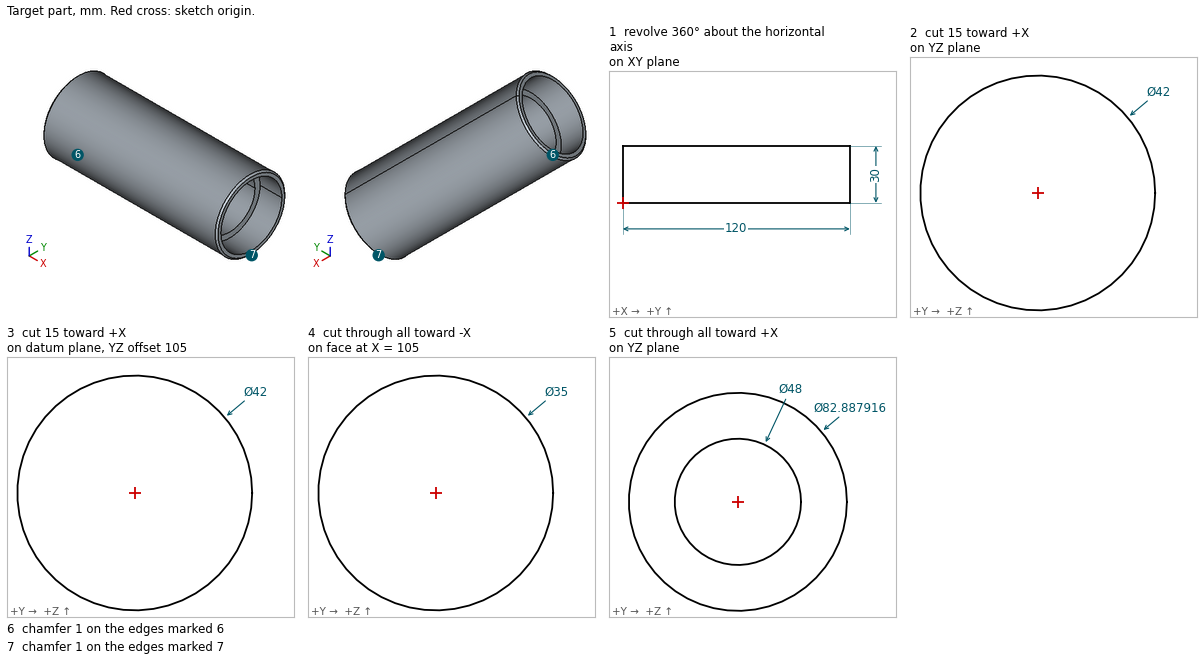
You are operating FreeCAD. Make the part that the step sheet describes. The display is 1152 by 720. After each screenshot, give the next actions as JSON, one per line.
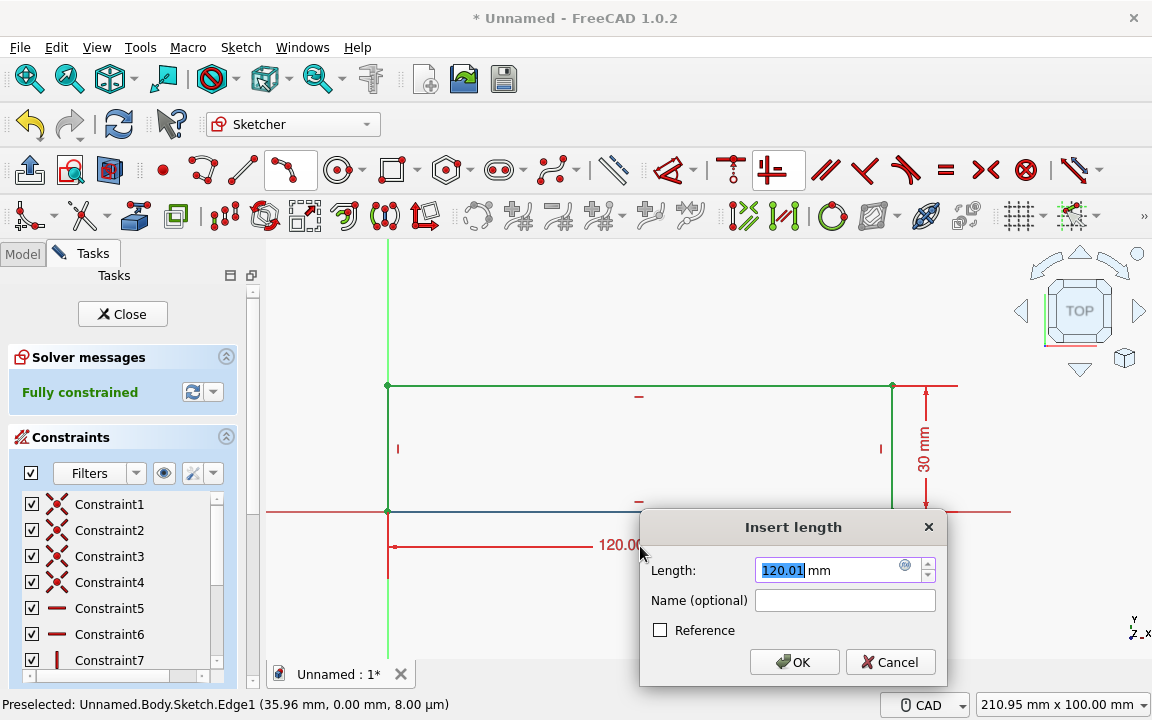
{"action": "type", "text": "120"}
{"action": "key", "text": "Return"}
{"action": "key", "text": "Escape"}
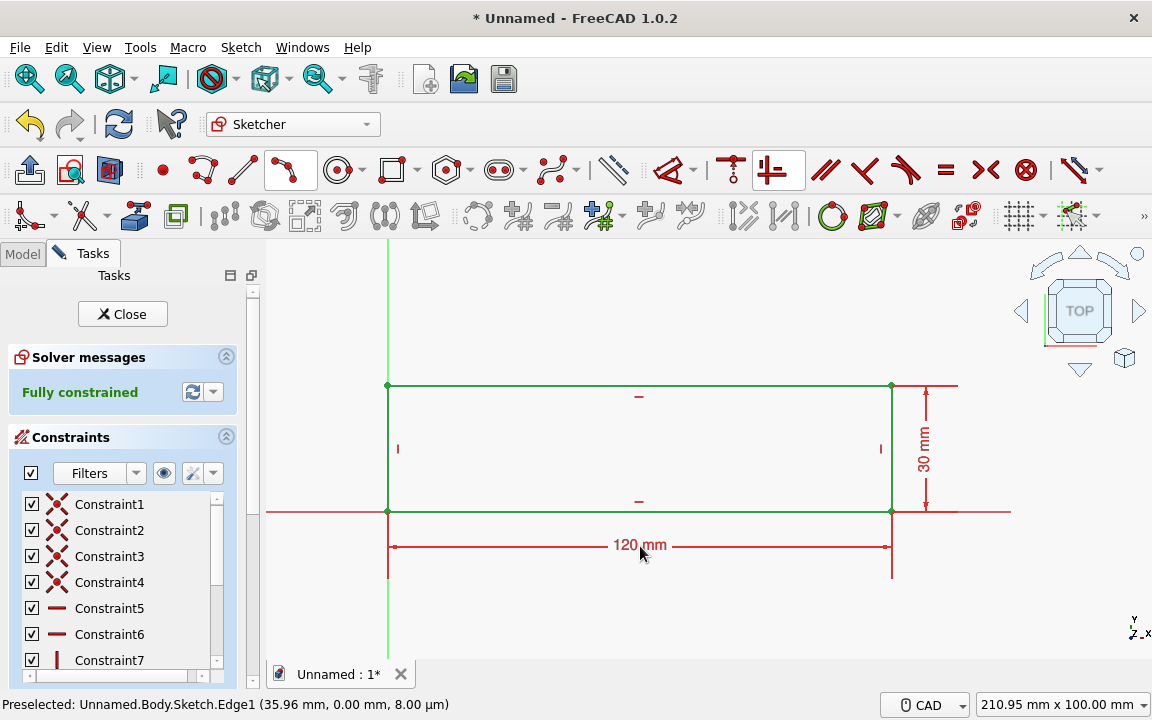
{"action": "left_click", "coordinate": [123, 314]}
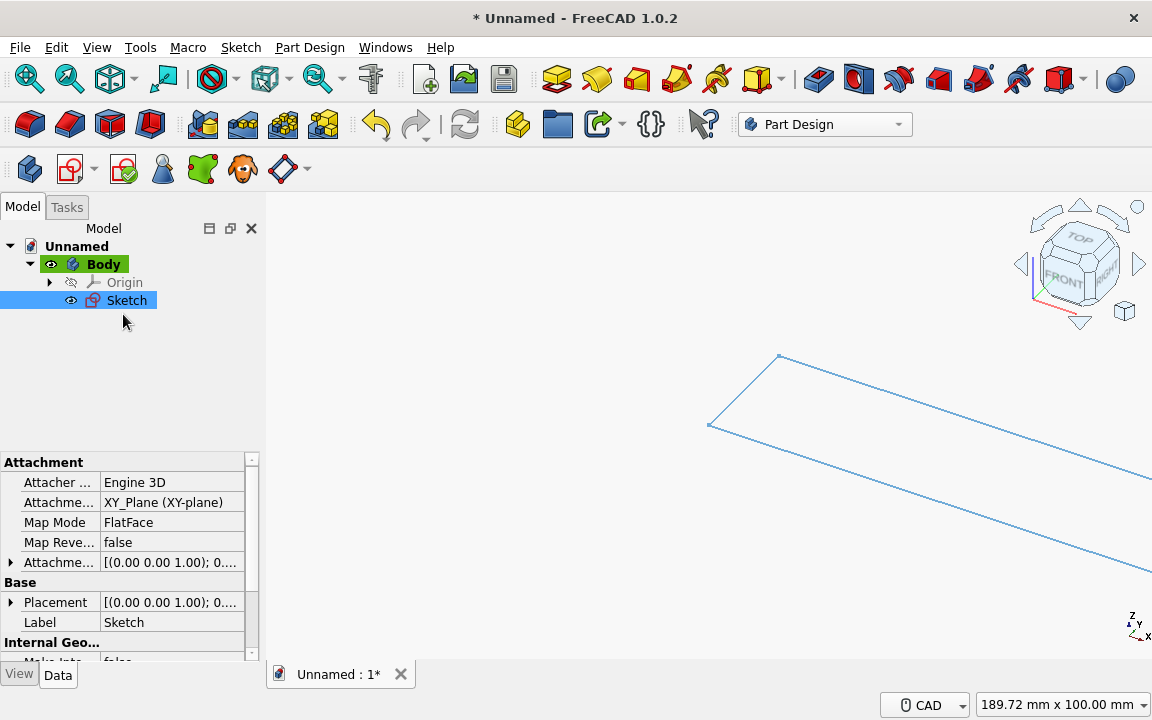
{"action": "left_click", "coordinate": [598, 80]}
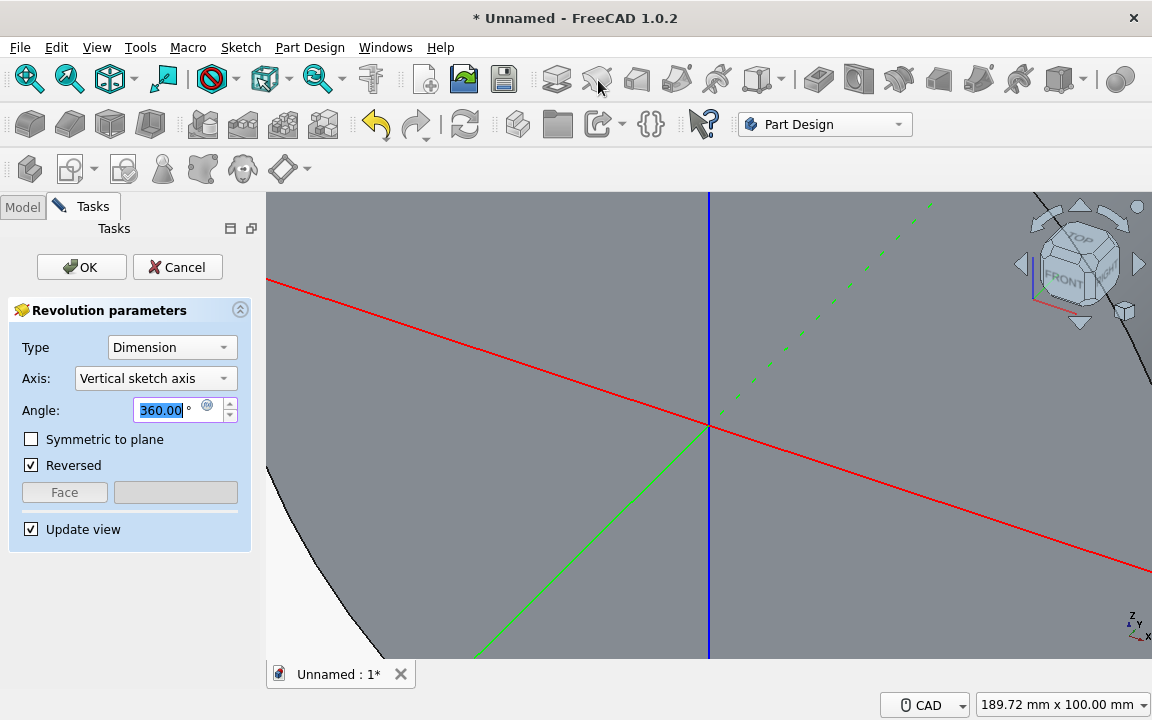
{"action": "left_click", "coordinate": [156, 378]}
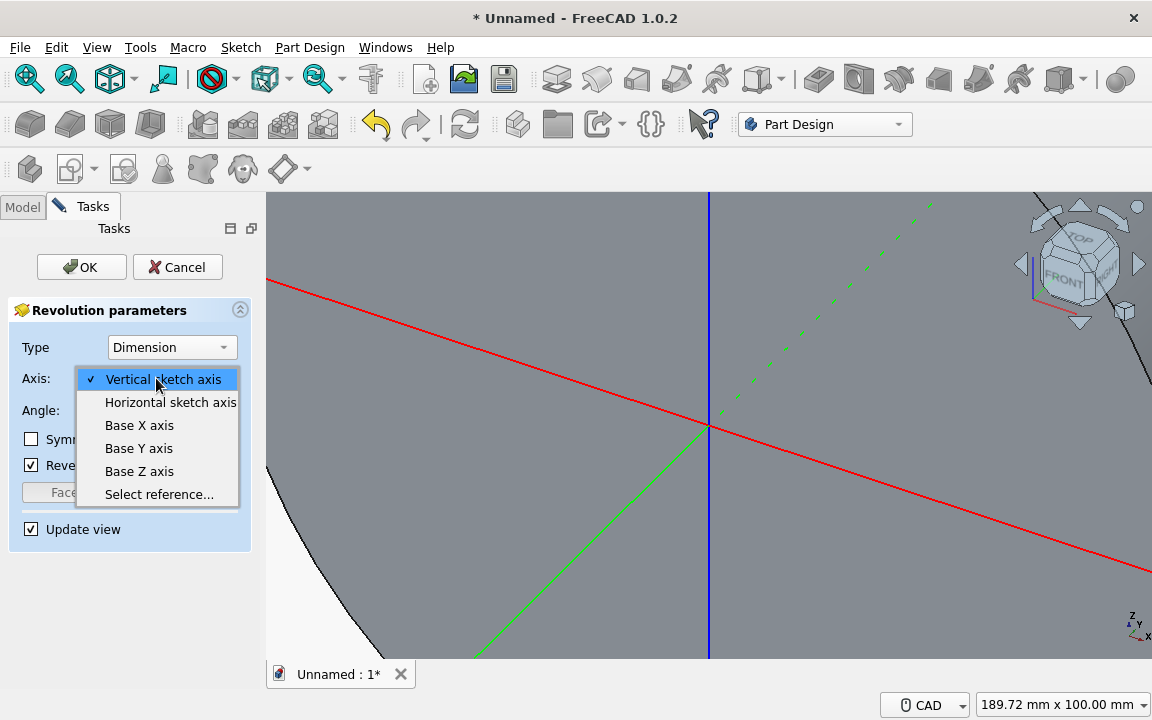
{"action": "left_click", "coordinate": [156, 402]}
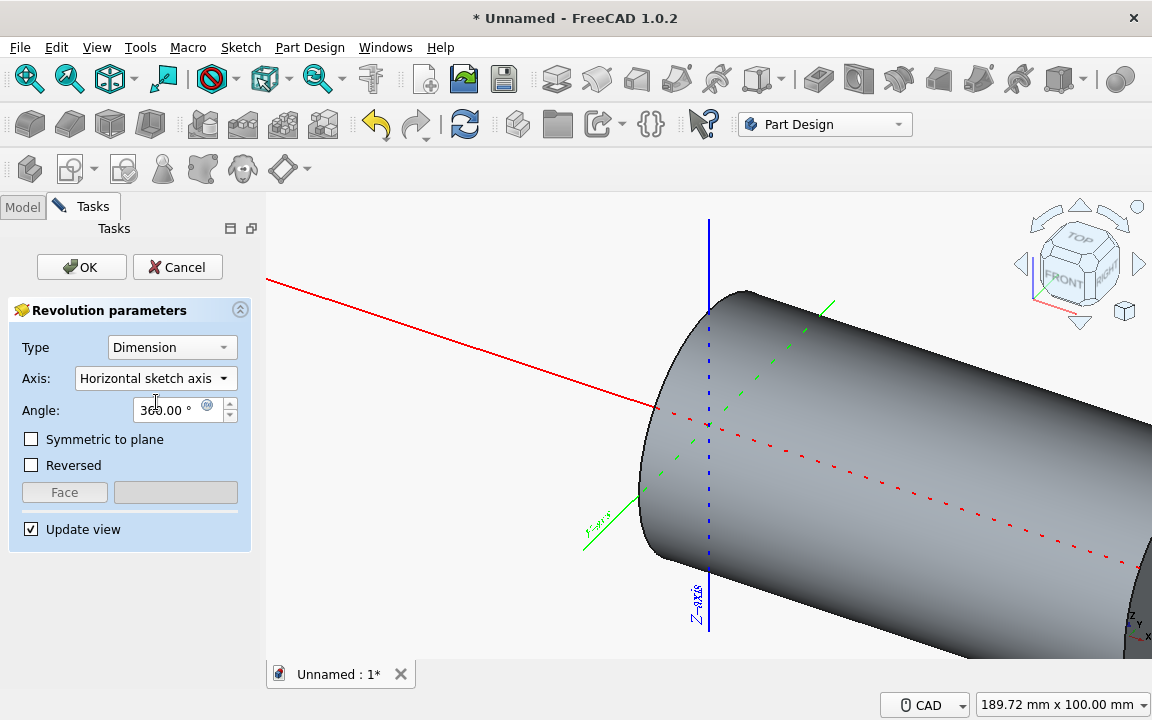
{"action": "left_click", "coordinate": [82, 267]}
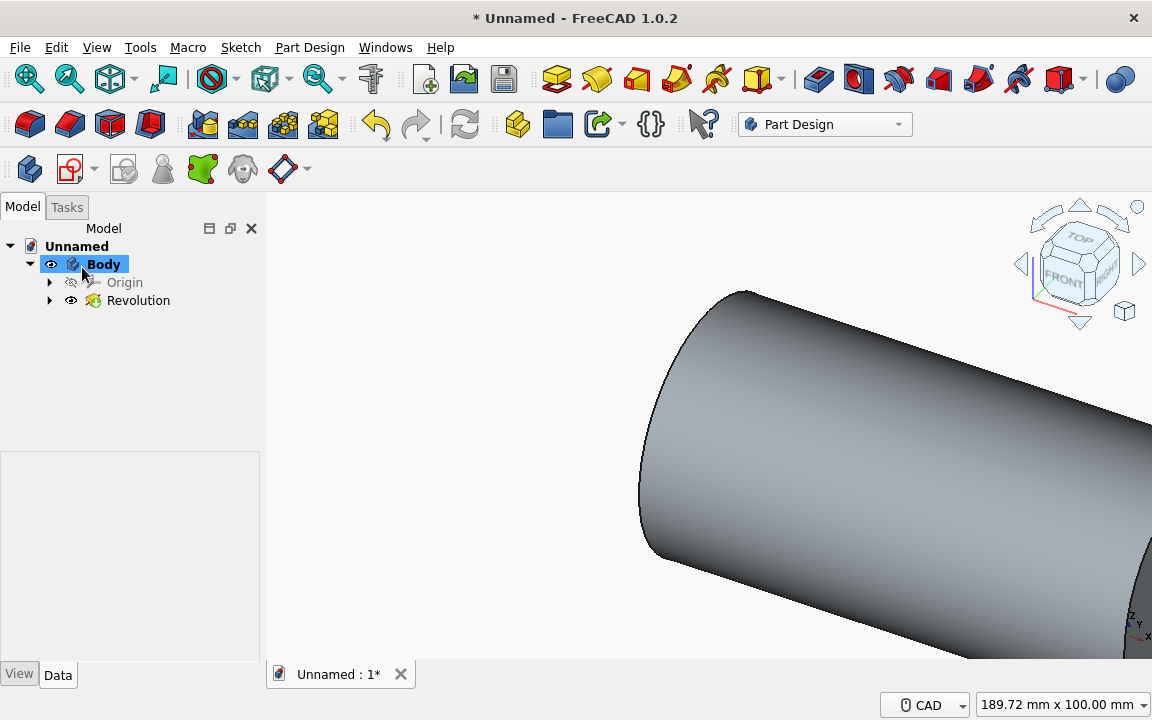
{"action": "key", "text": "v f"}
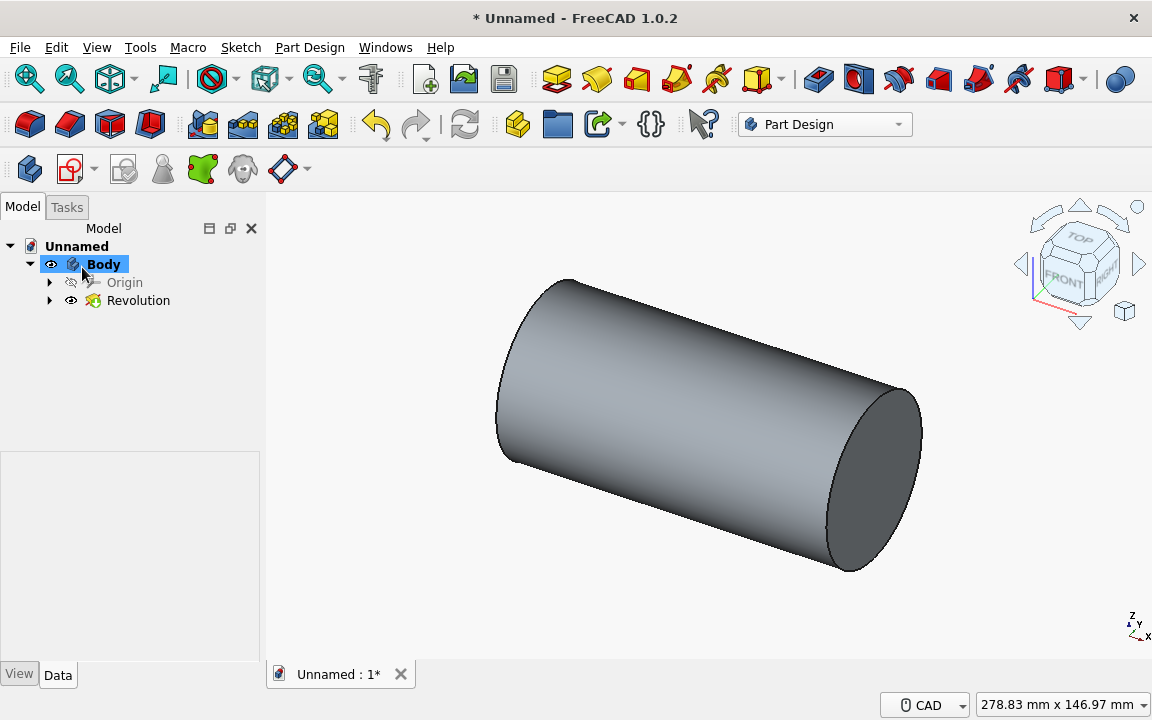
{"action": "left_click", "coordinate": [70, 170]}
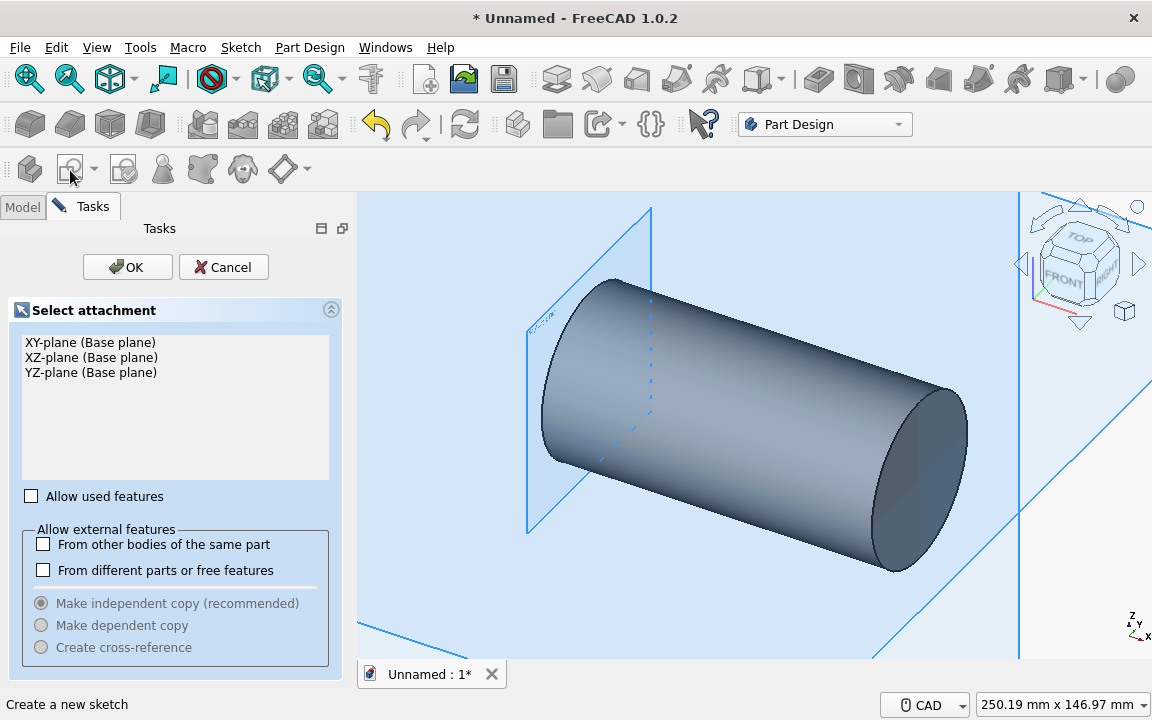
{"action": "left_click", "coordinate": [82, 372]}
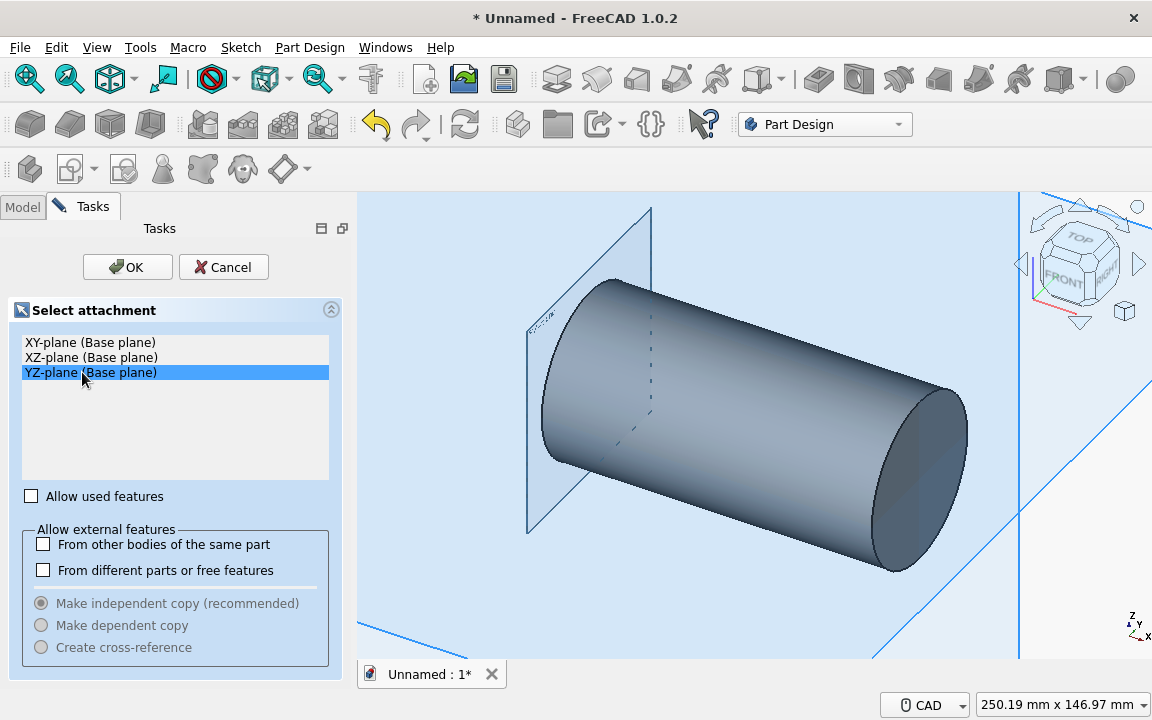
{"action": "left_click", "coordinate": [128, 267]}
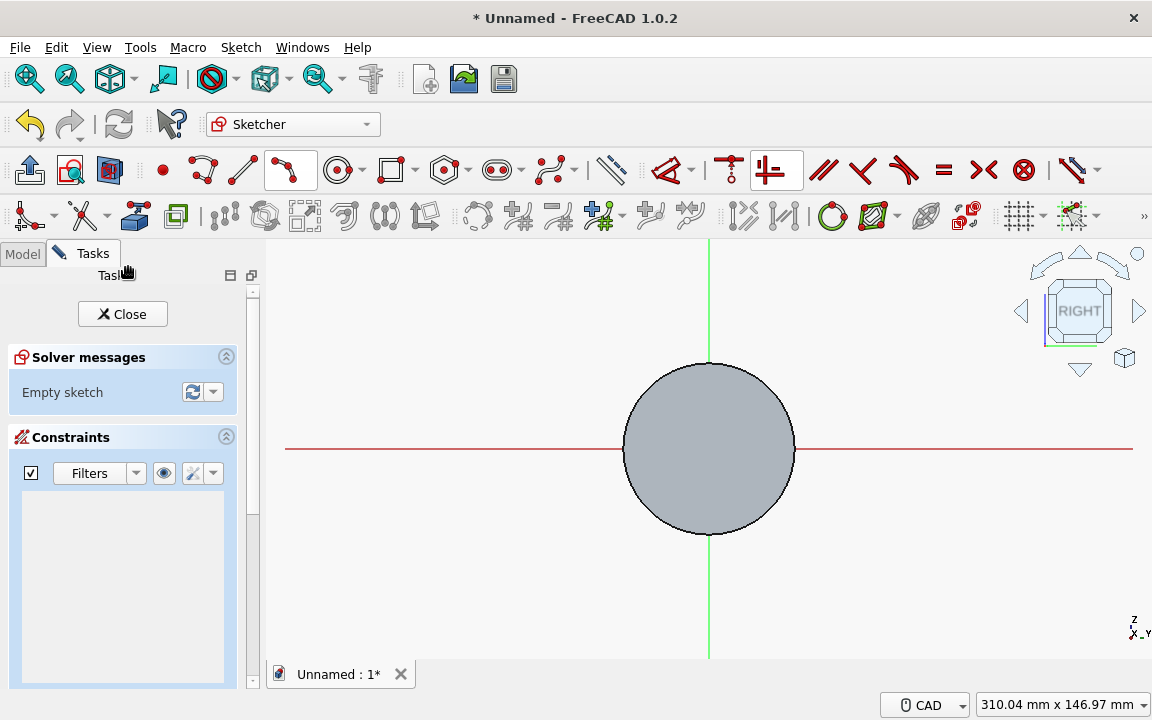
{"action": "key", "text": "q s"}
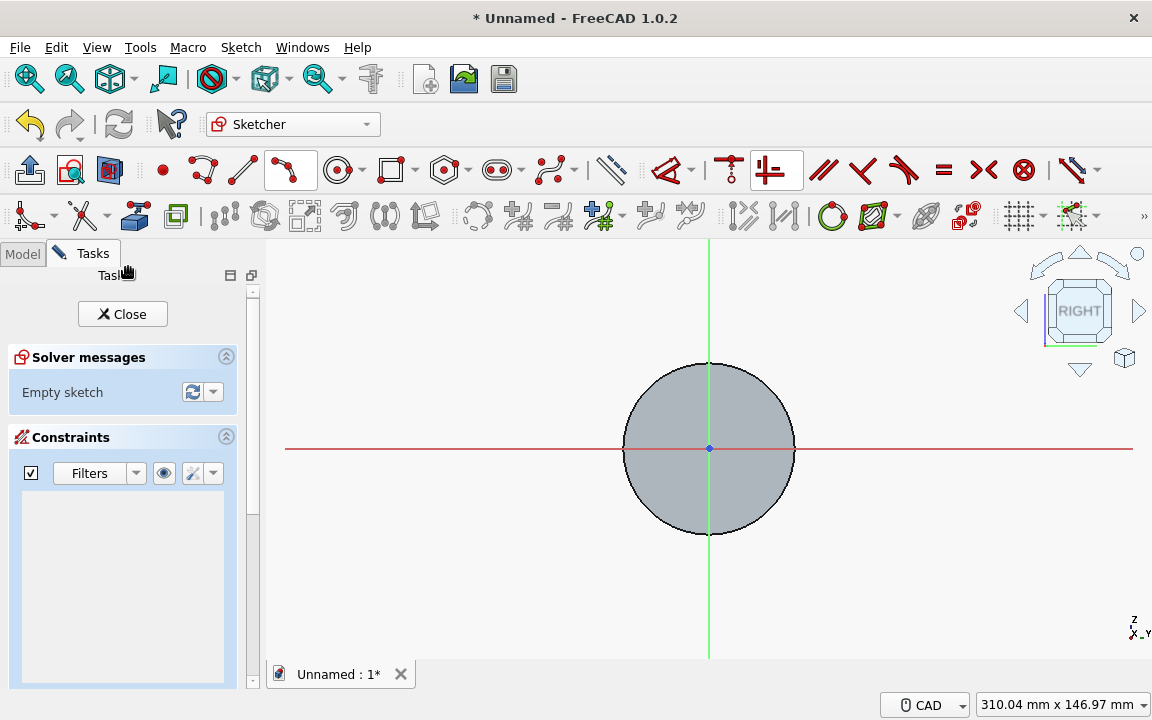
{"action": "scroll", "coordinate": [765, 449], "scroll_direction": "up", "scroll_amount": 4}